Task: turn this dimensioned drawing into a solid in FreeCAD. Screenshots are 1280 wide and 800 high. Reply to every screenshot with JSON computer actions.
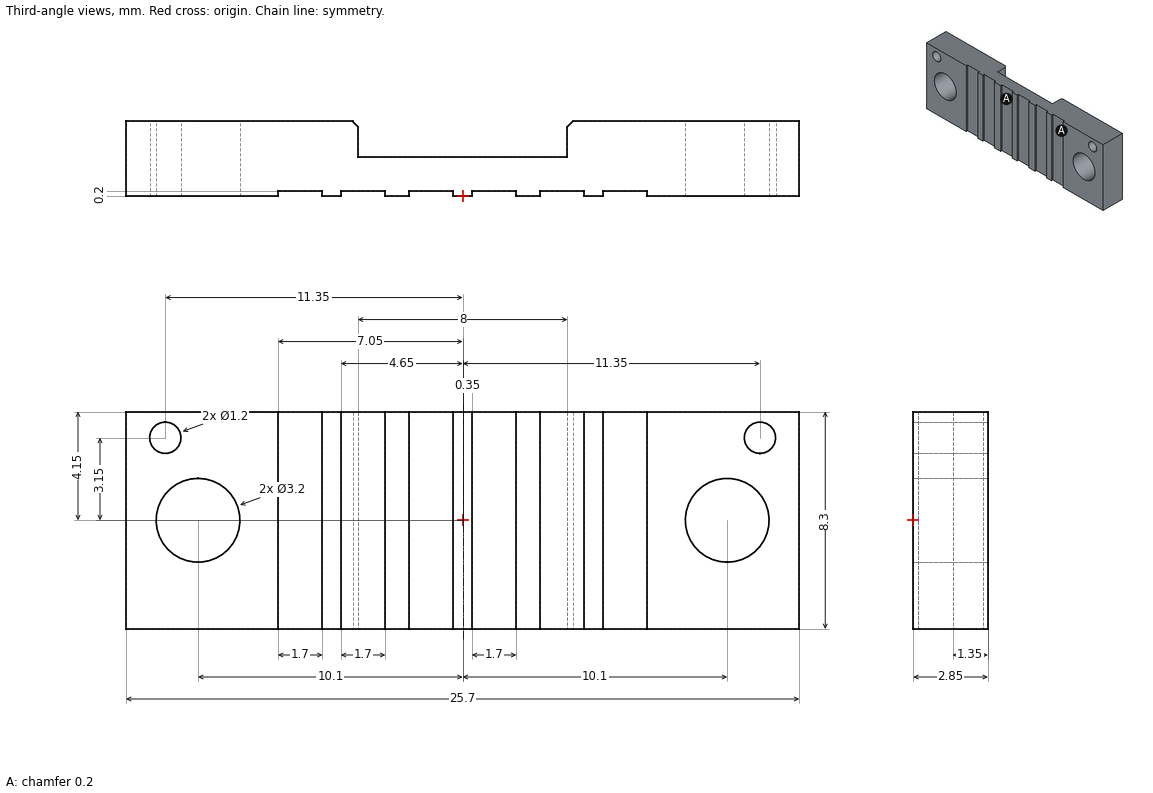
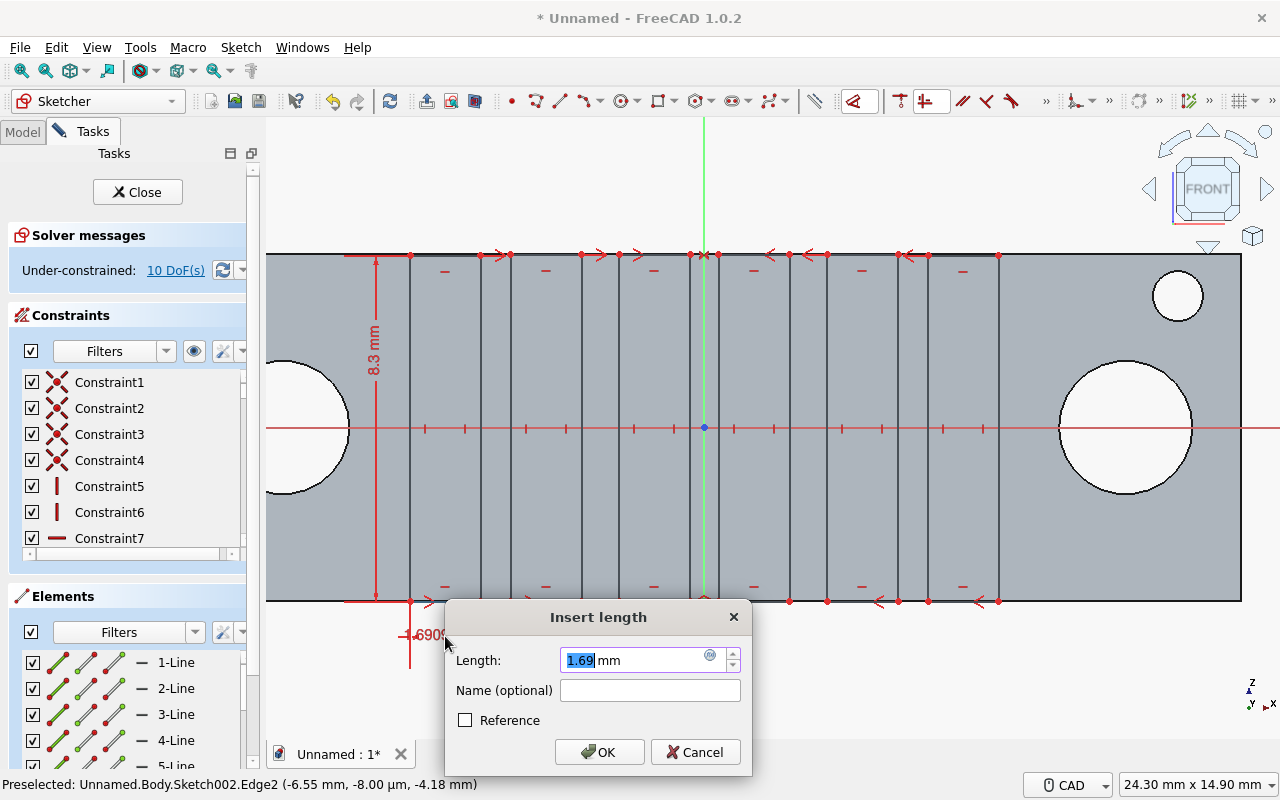
{"action": "type", "text": "1.7"}
{"action": "key", "text": "Return"}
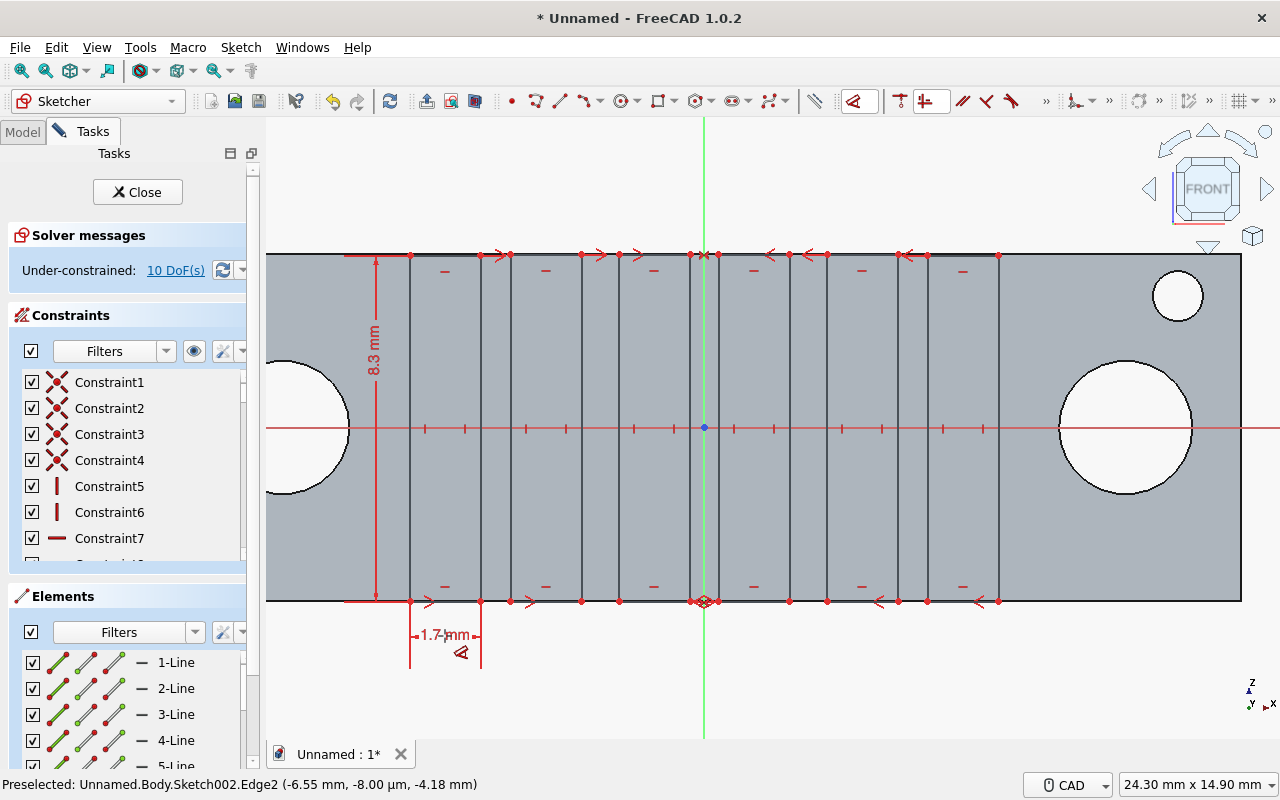
{"action": "left_click", "coordinate": [719, 359]}
{"action": "left_click", "coordinate": [753, 349]}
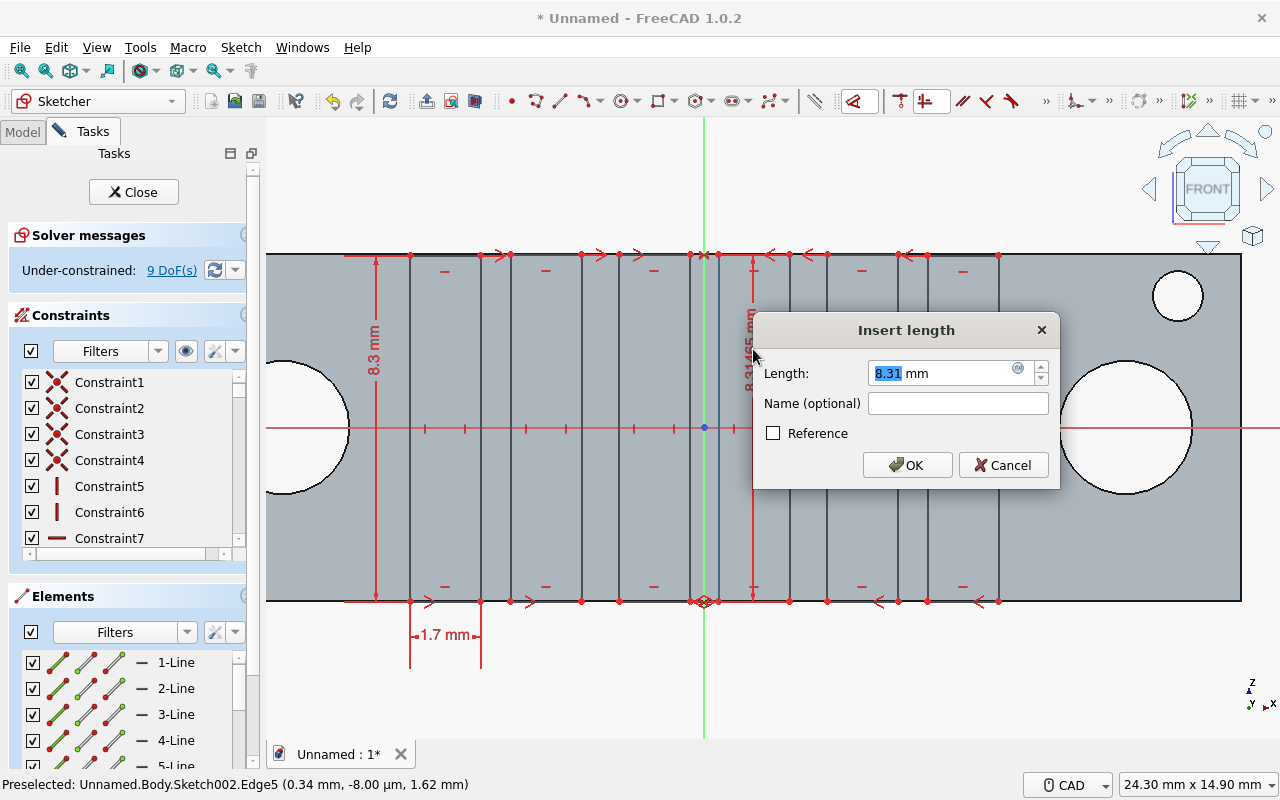
{"action": "type", "text": "8.3"}
{"action": "key", "text": "Return"}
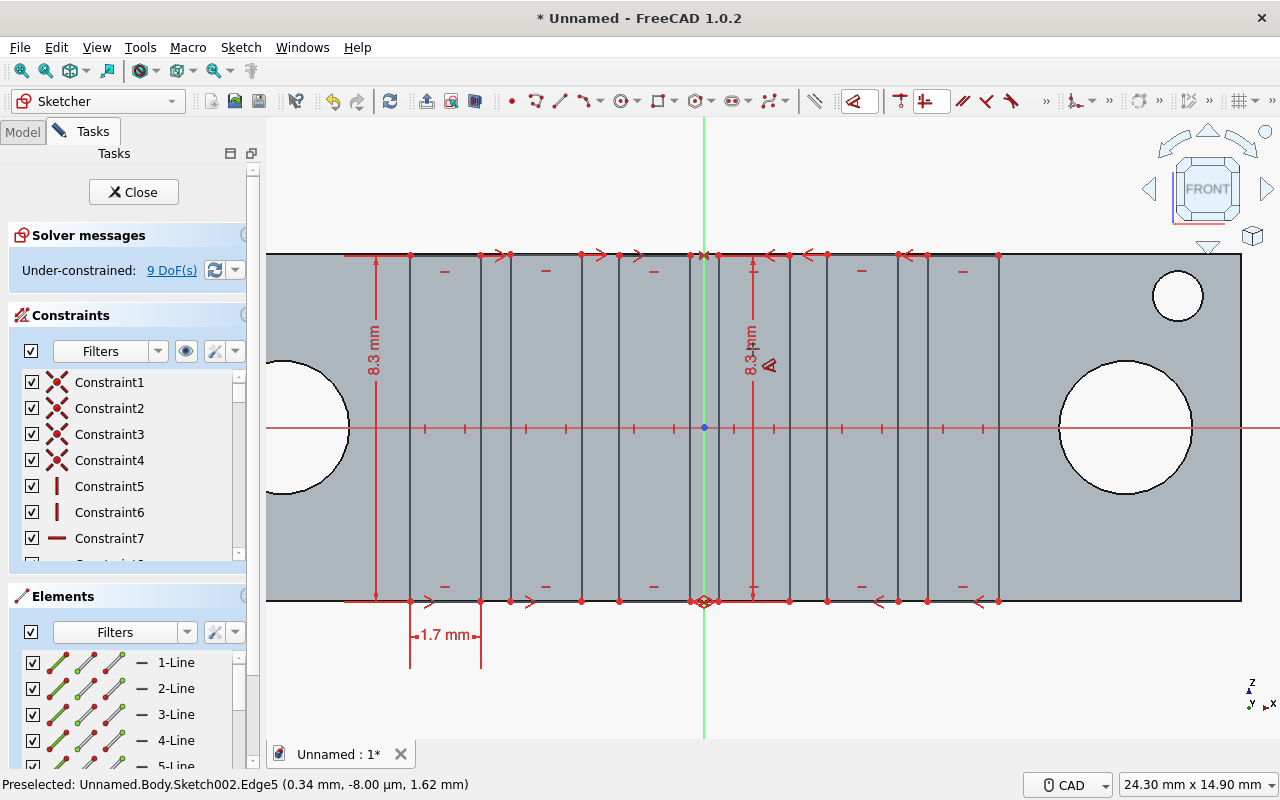
{"action": "left_click", "coordinate": [740, 602]}
{"action": "left_click", "coordinate": [754, 636]}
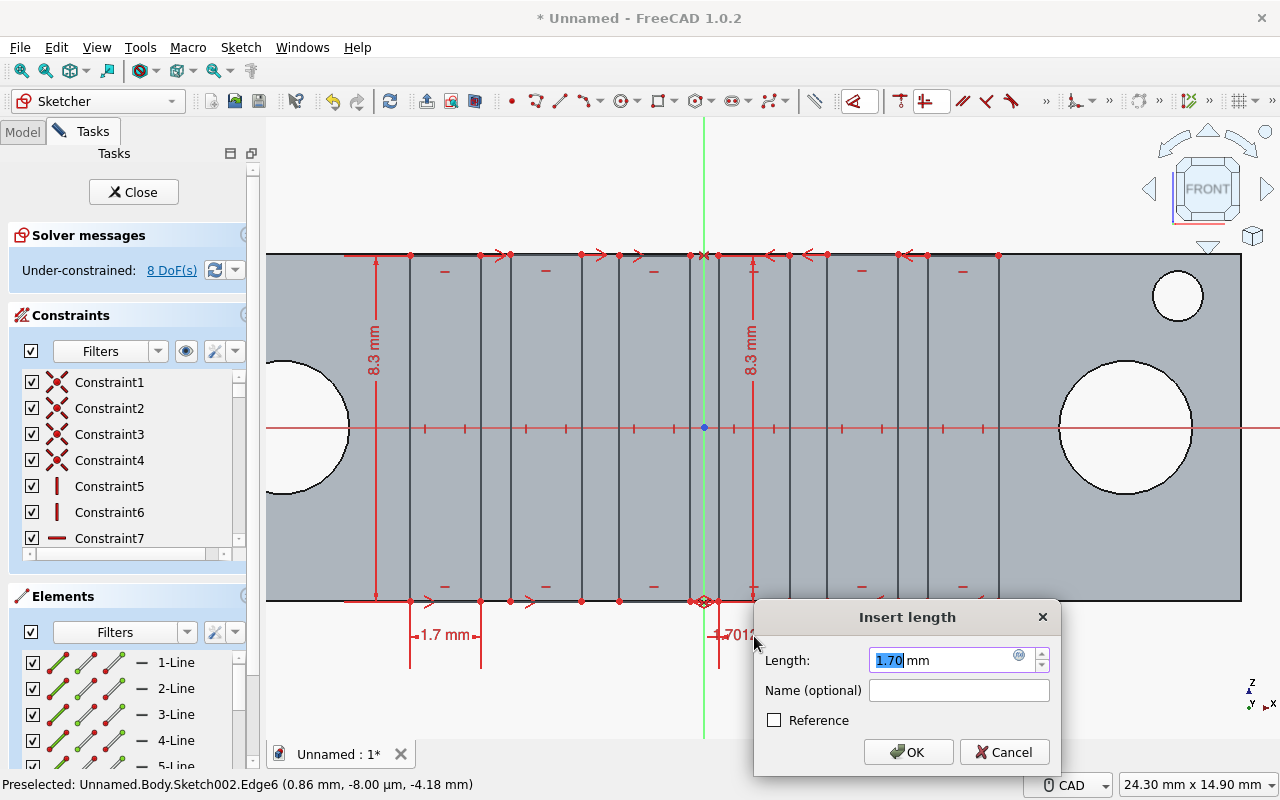
{"action": "type", "text": "1.7"}
{"action": "key", "text": "Return"}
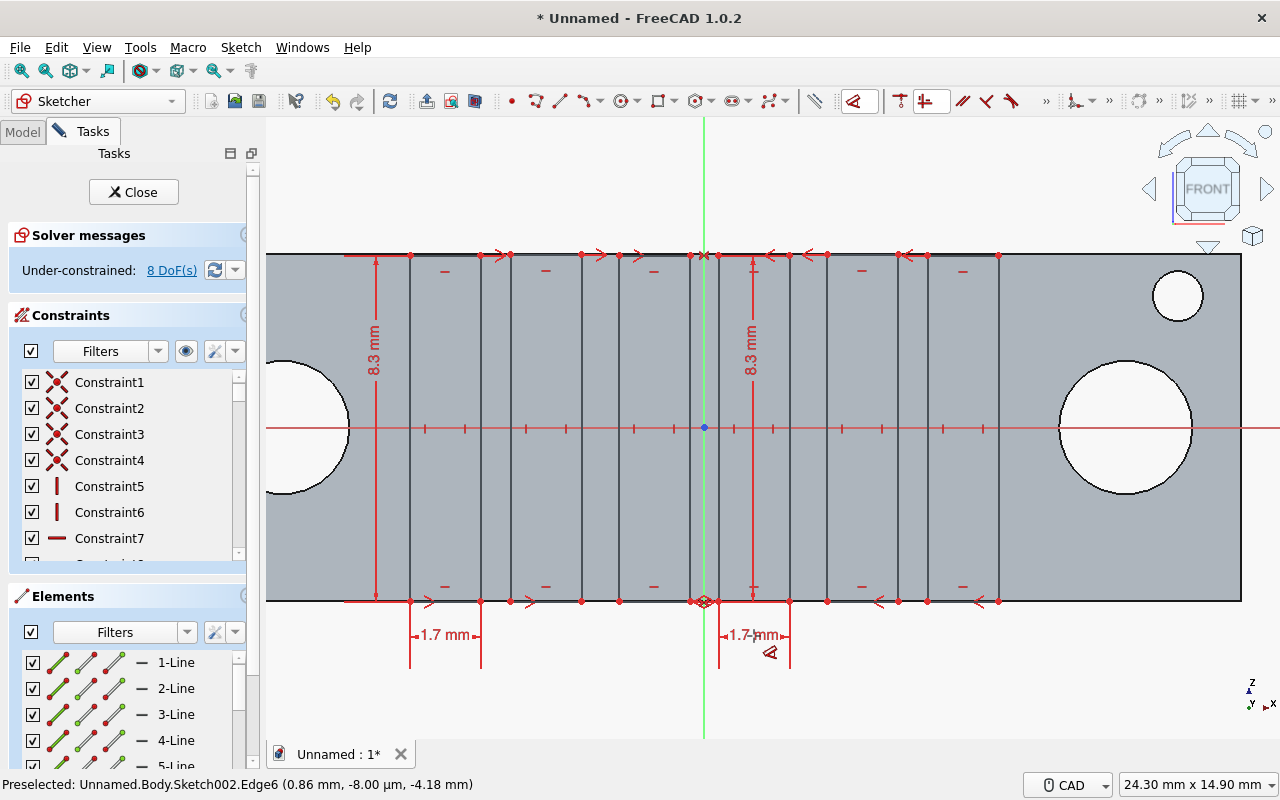
{"action": "left_click", "coordinate": [511, 359]}
{"action": "left_click", "coordinate": [545, 349]}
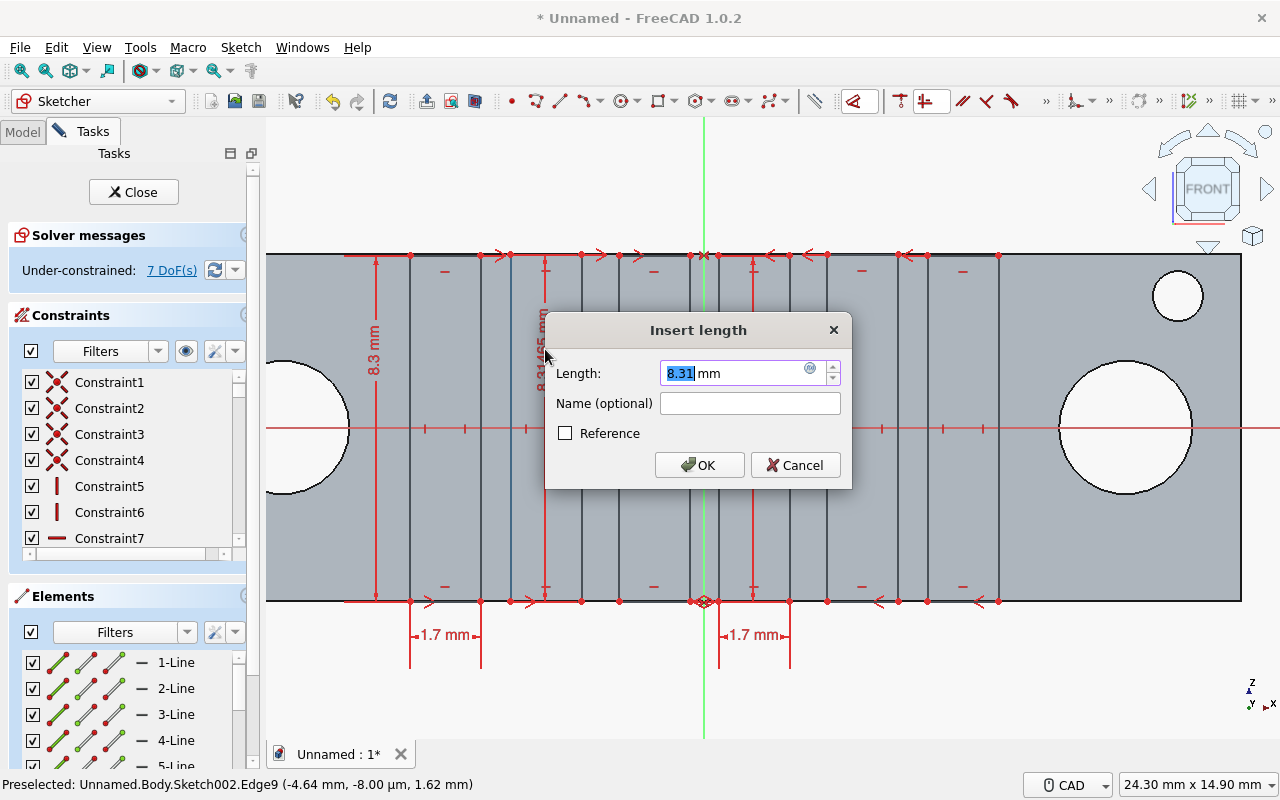
{"action": "type", "text": "8.3"}
{"action": "key", "text": "Return"}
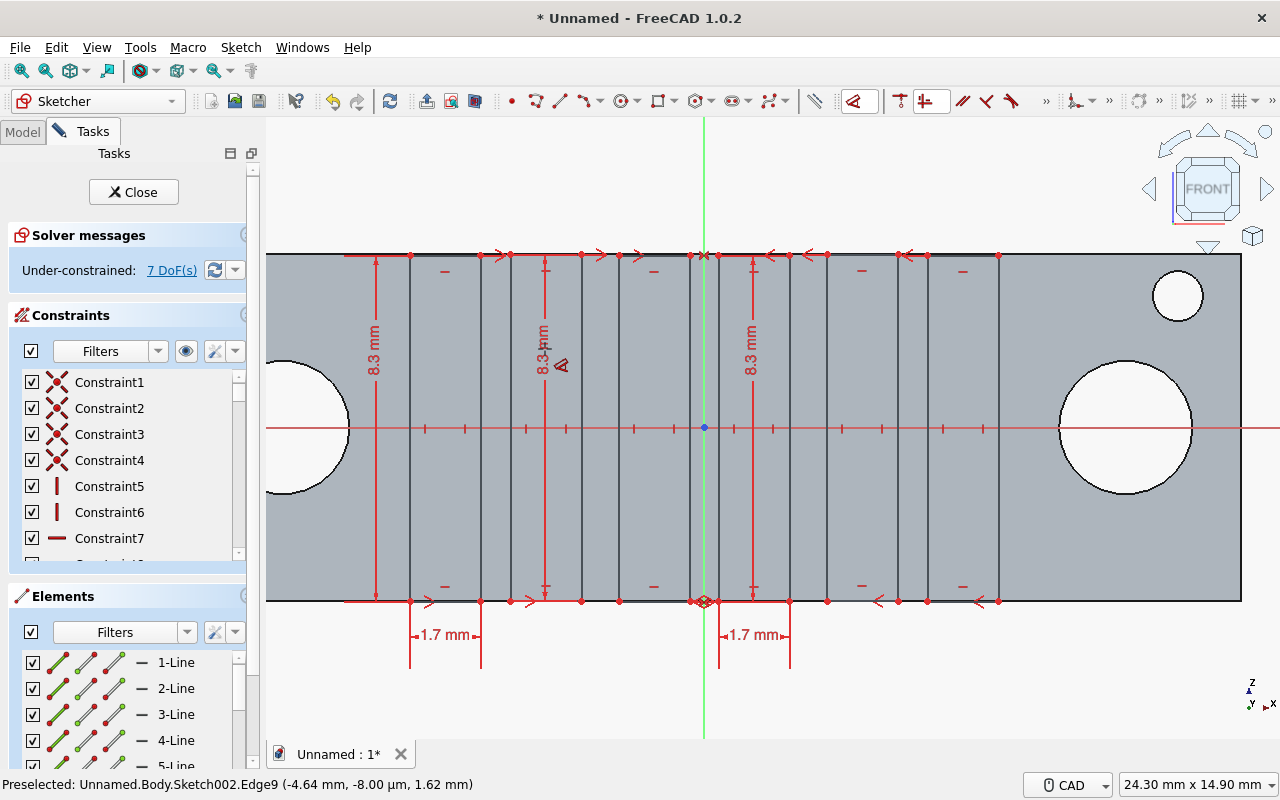
{"action": "left_click", "coordinate": [532, 601]}
{"action": "left_click", "coordinate": [546, 635]}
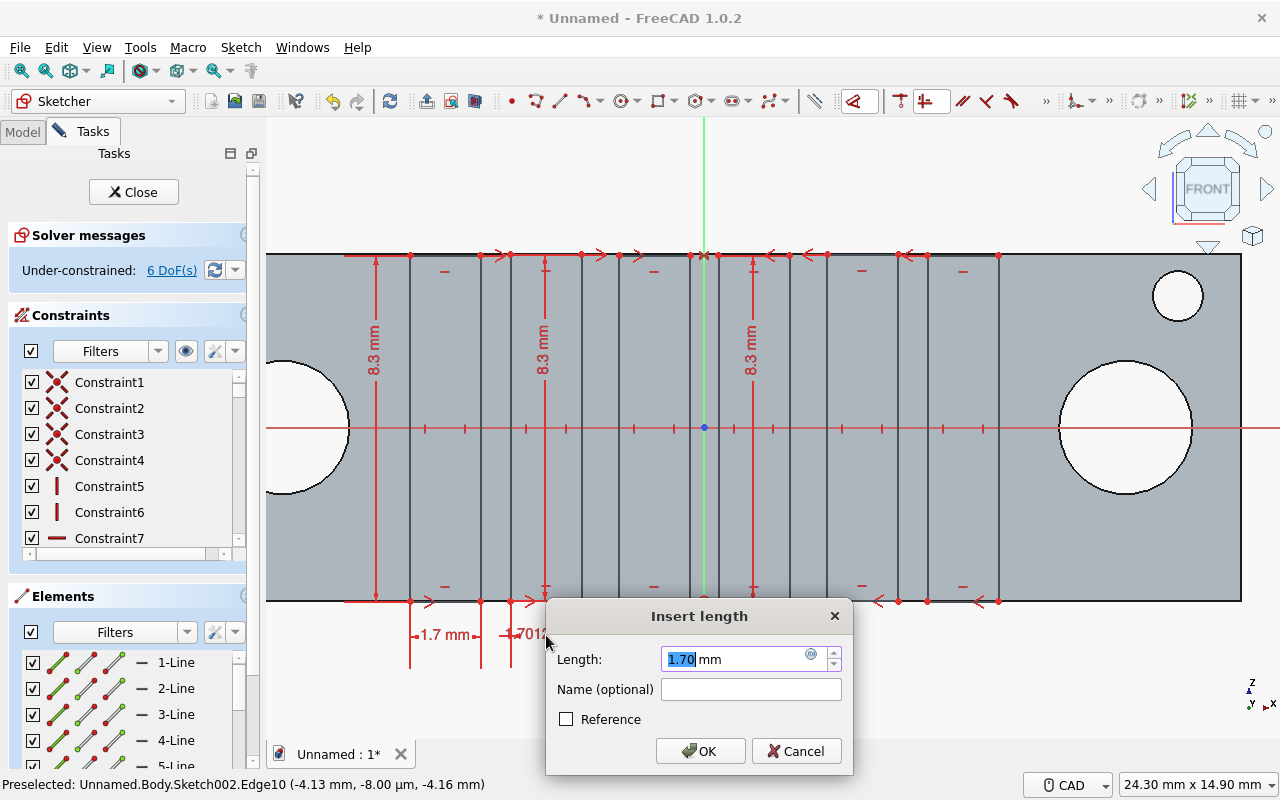
{"action": "type", "text": "1.7"}
{"action": "key", "text": "Return"}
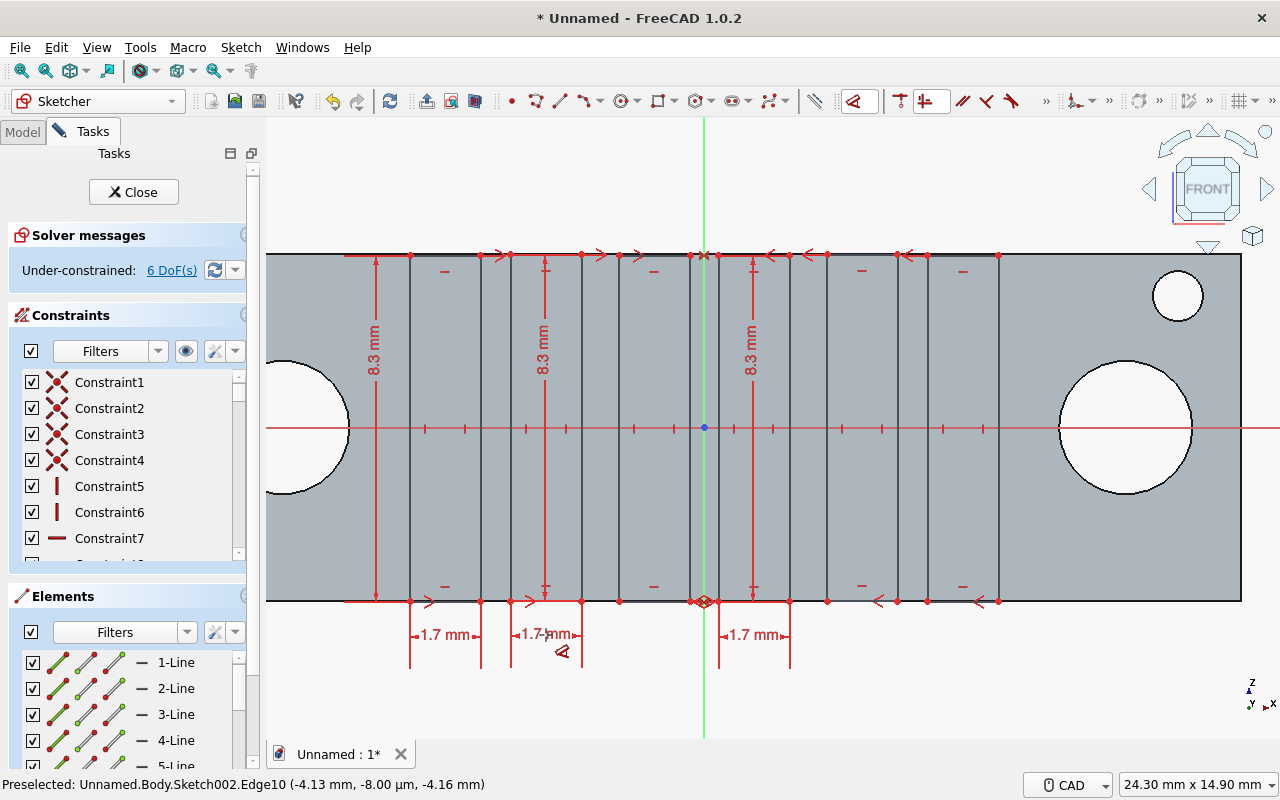
{"action": "left_click", "coordinate": [410, 256]}
{"action": "left_click", "coordinate": [557, 222]}